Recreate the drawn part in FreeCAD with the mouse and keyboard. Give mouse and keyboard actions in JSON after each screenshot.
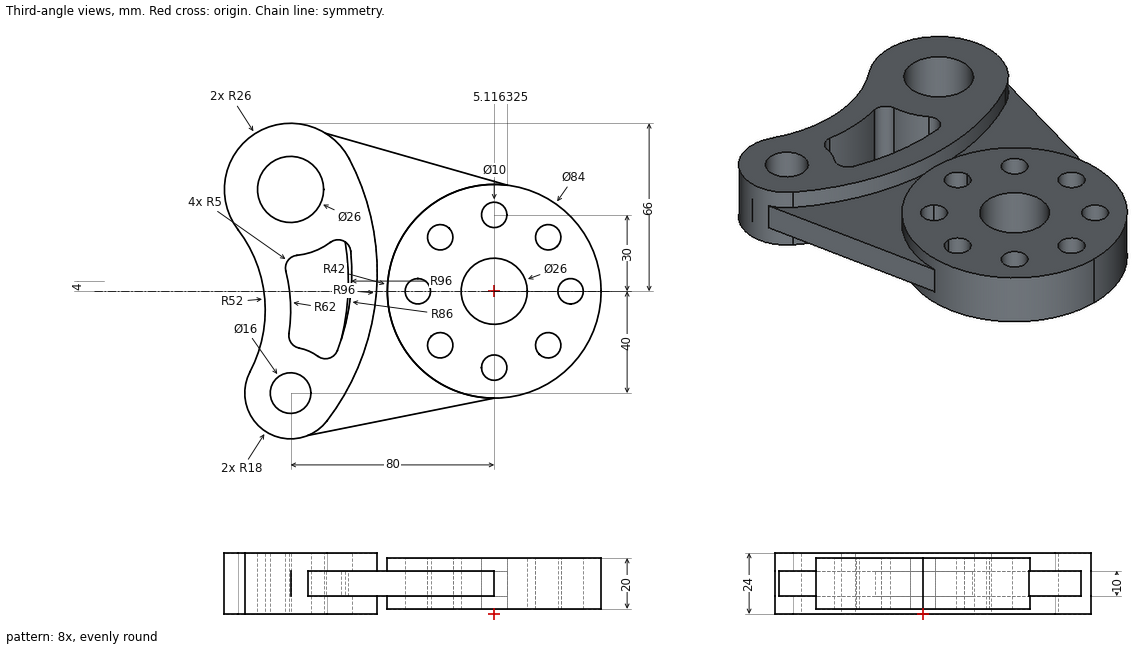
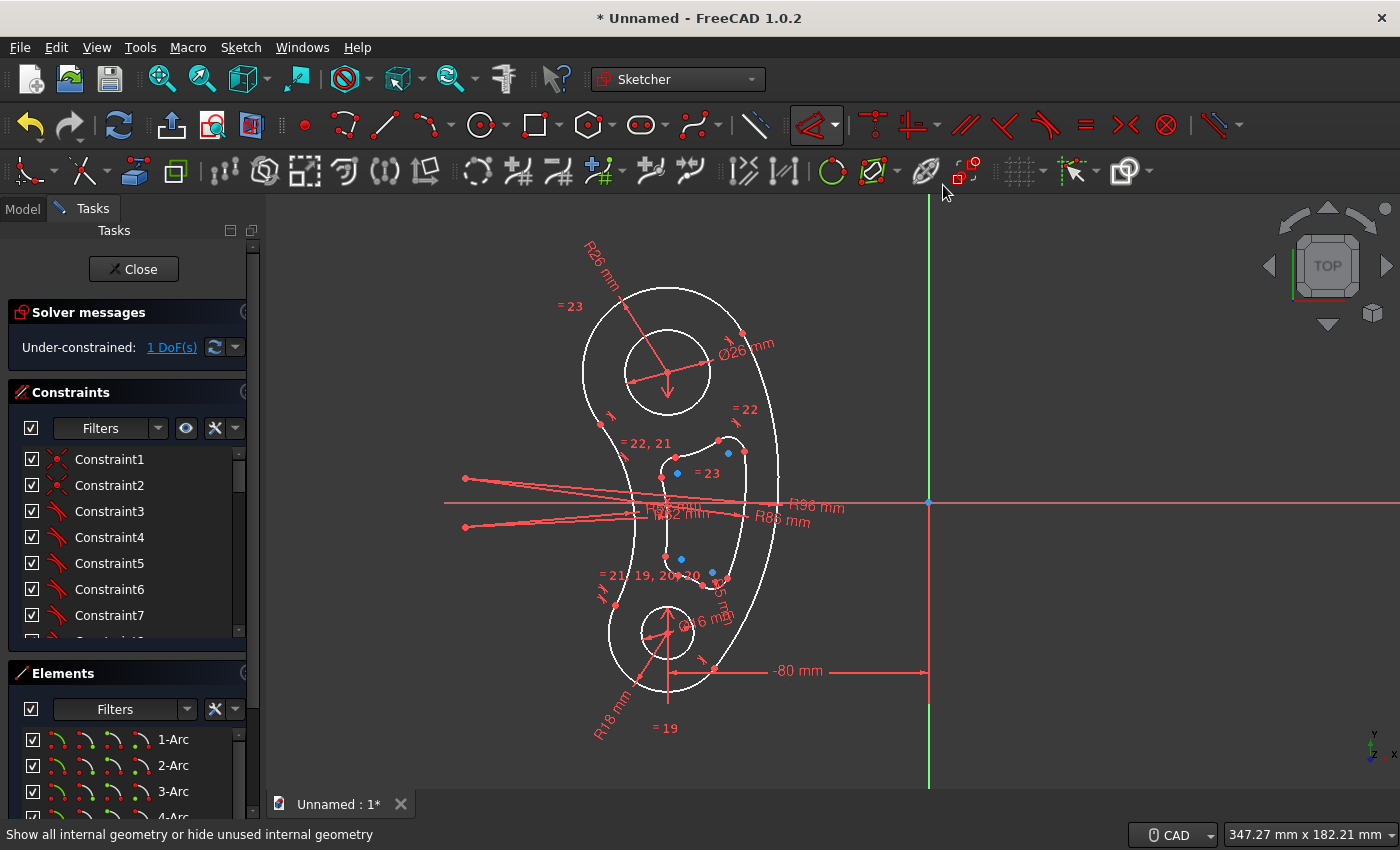
{"action": "left_click", "coordinate": [668, 633]}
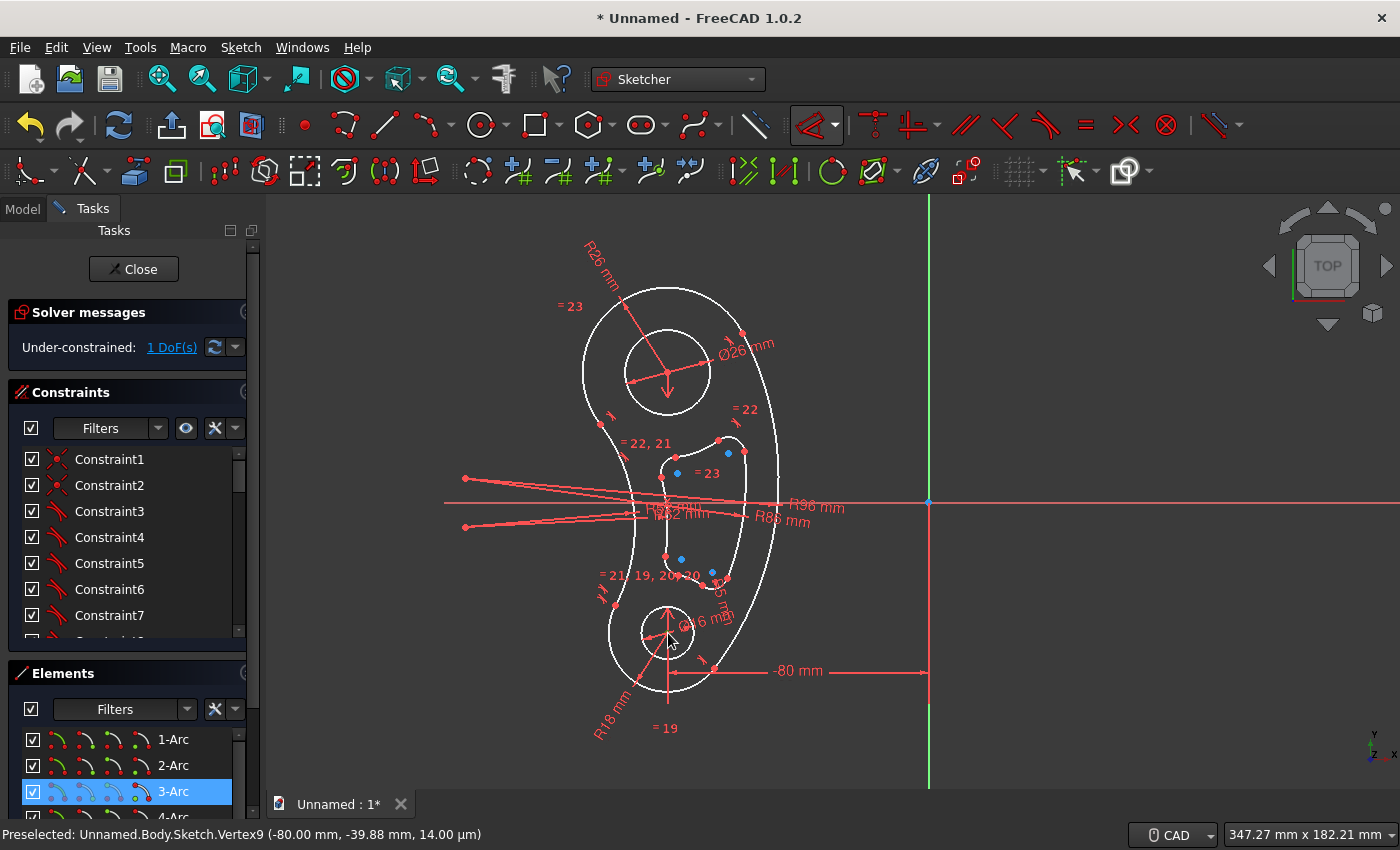
{"action": "left_click", "coordinate": [838, 126]}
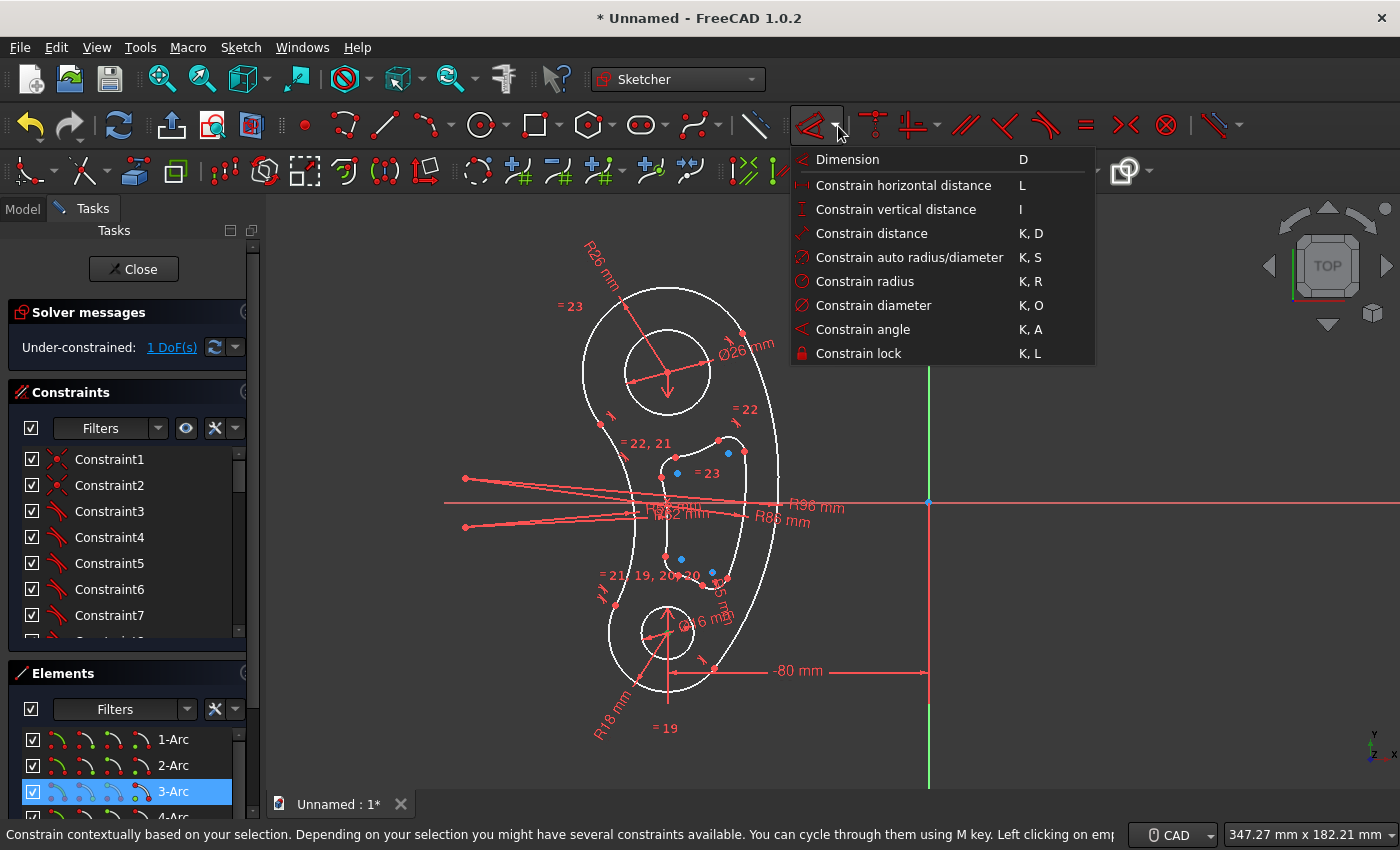
{"action": "left_click", "coordinate": [943, 209]}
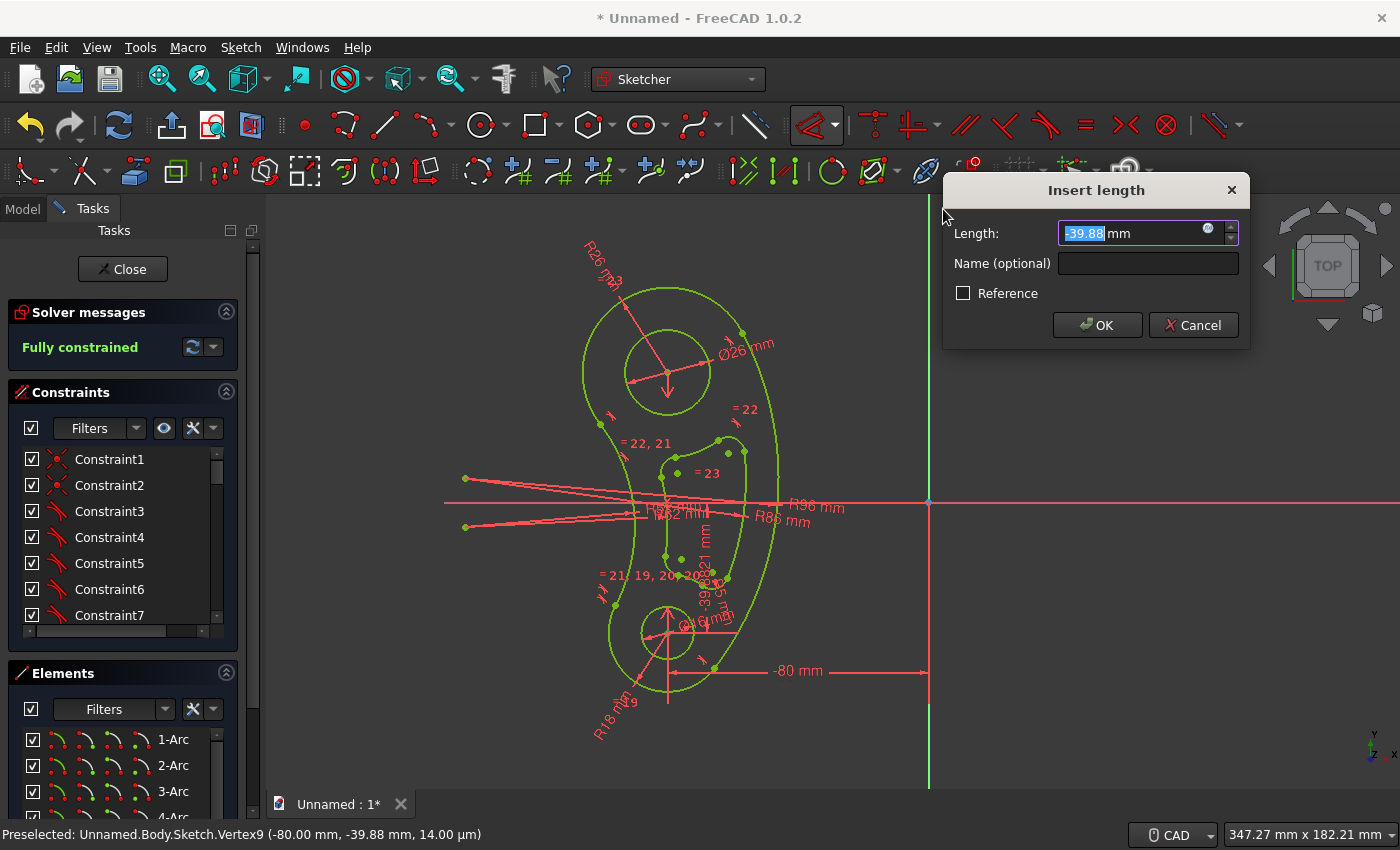
{"action": "type", "text": "-40"}
{"action": "key", "text": "Return"}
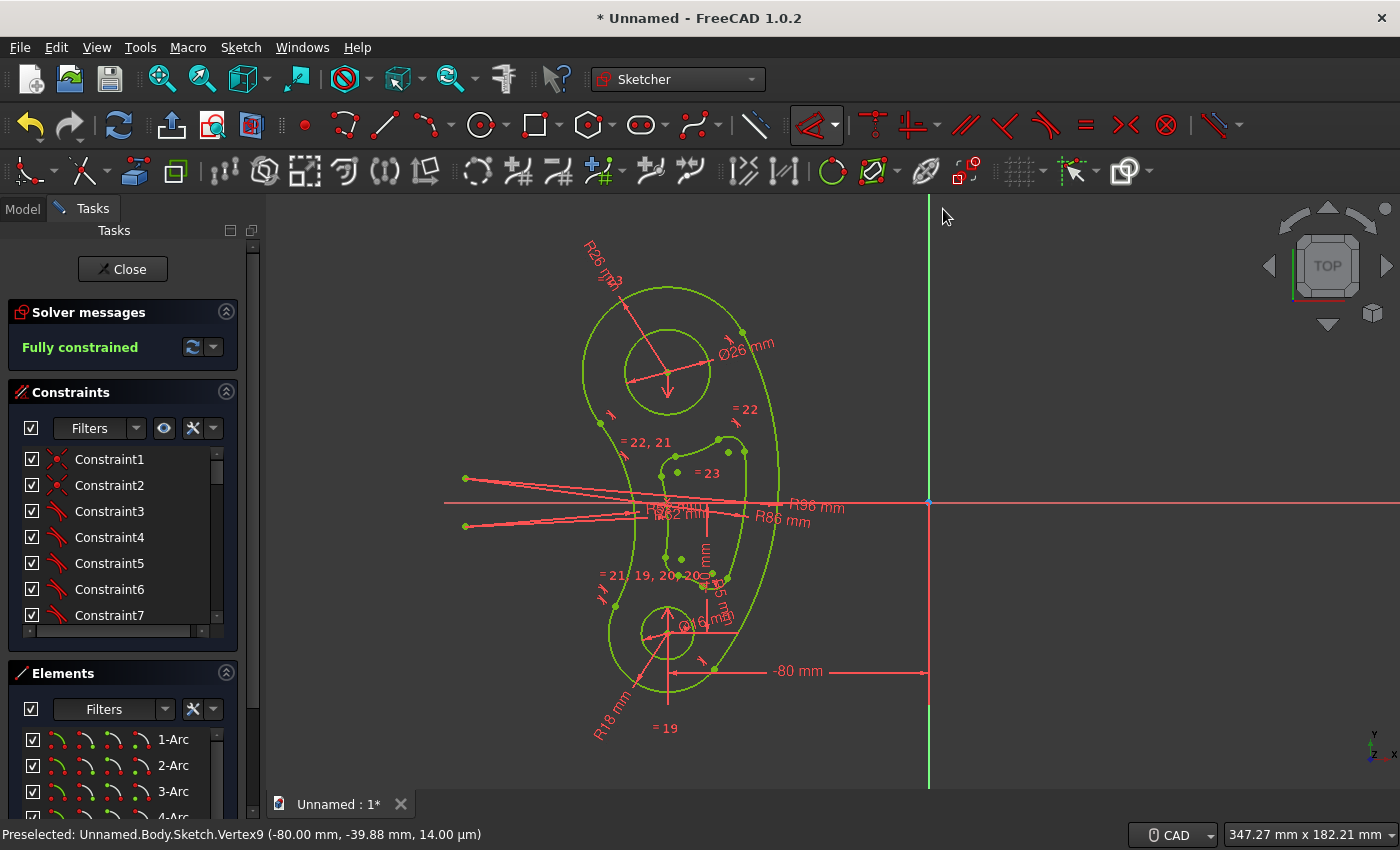
{"action": "left_click", "coordinate": [123, 269]}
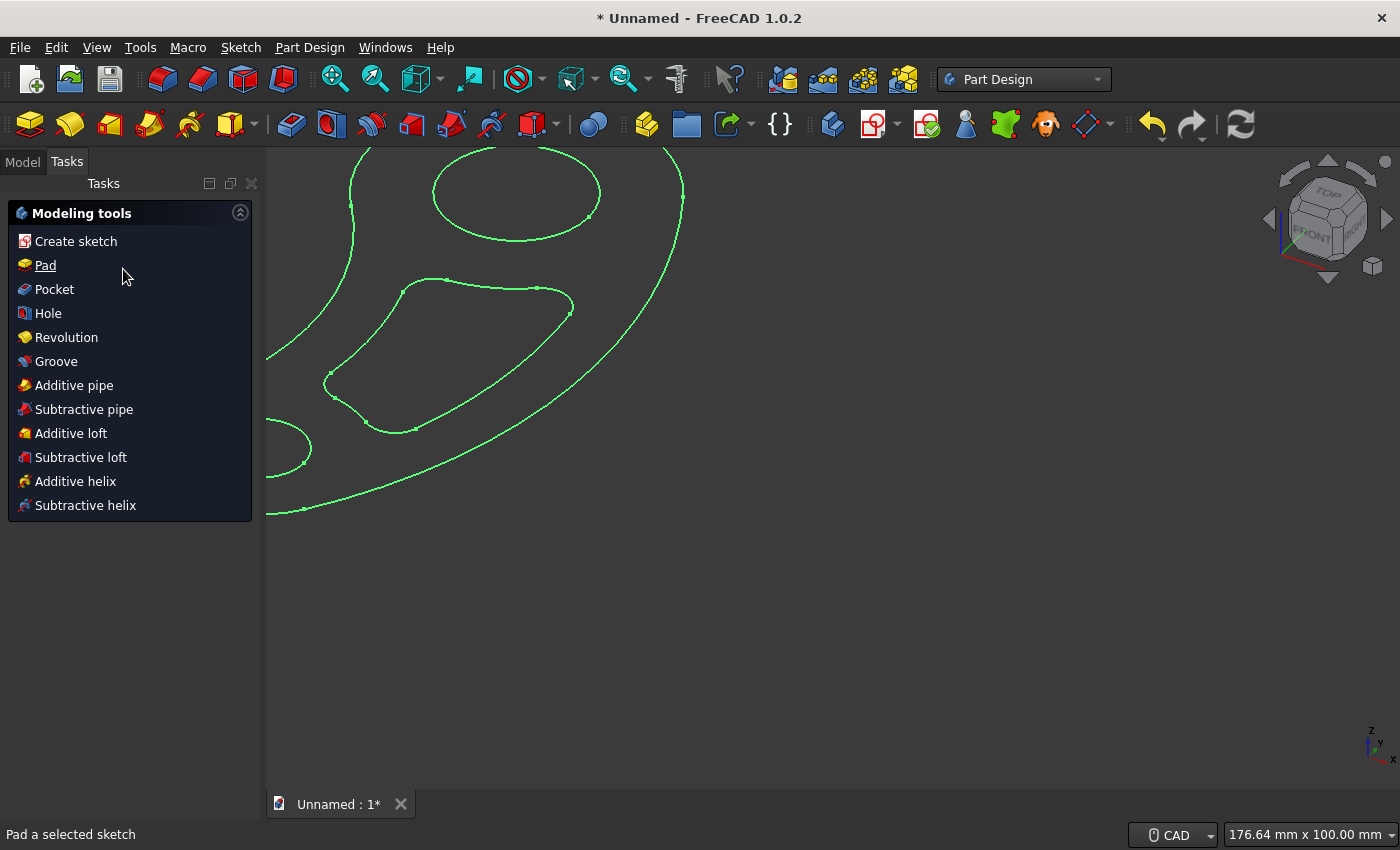
{"action": "left_click", "coordinate": [30, 124]}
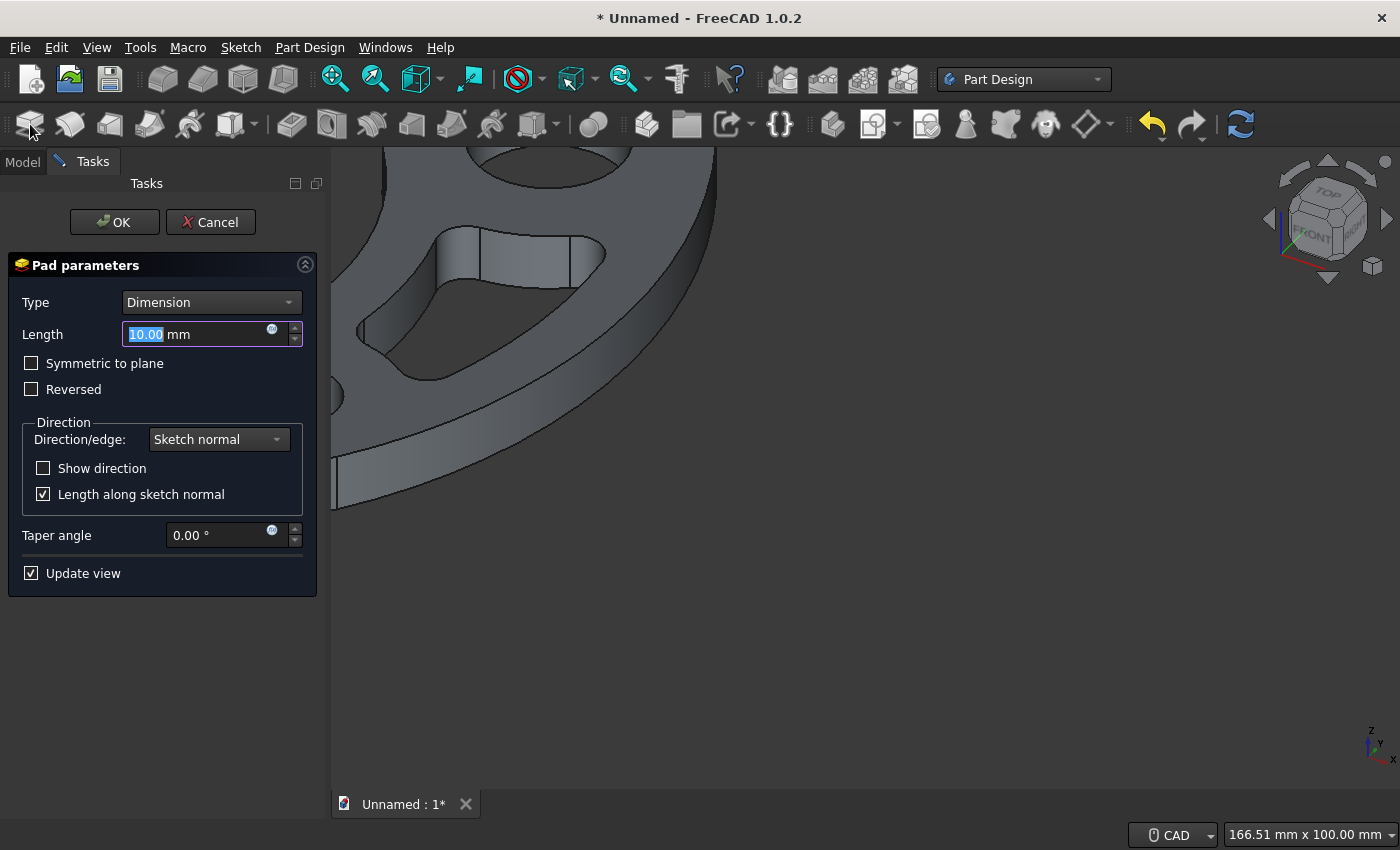
{"action": "type", "text": "24"}
{"action": "key", "text": "Tab"}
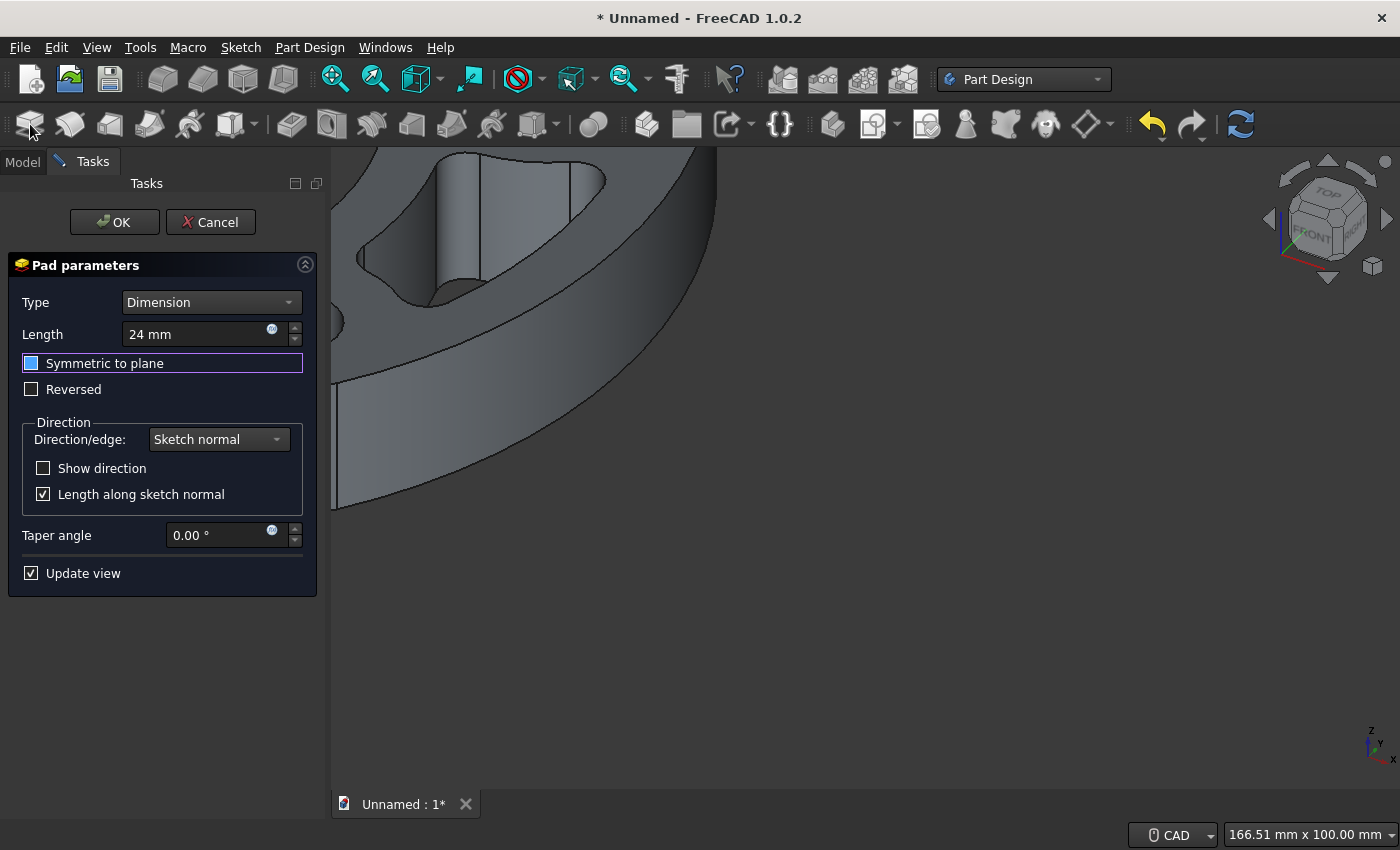
{"action": "left_click", "coordinate": [115, 222]}